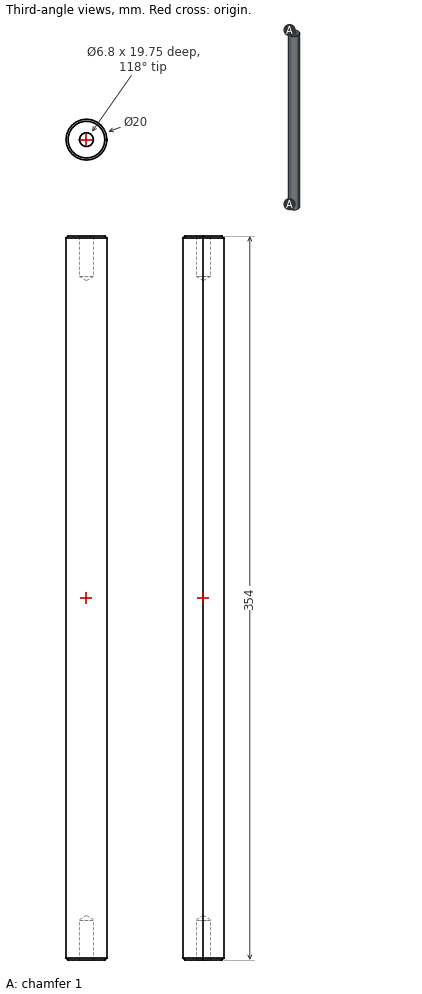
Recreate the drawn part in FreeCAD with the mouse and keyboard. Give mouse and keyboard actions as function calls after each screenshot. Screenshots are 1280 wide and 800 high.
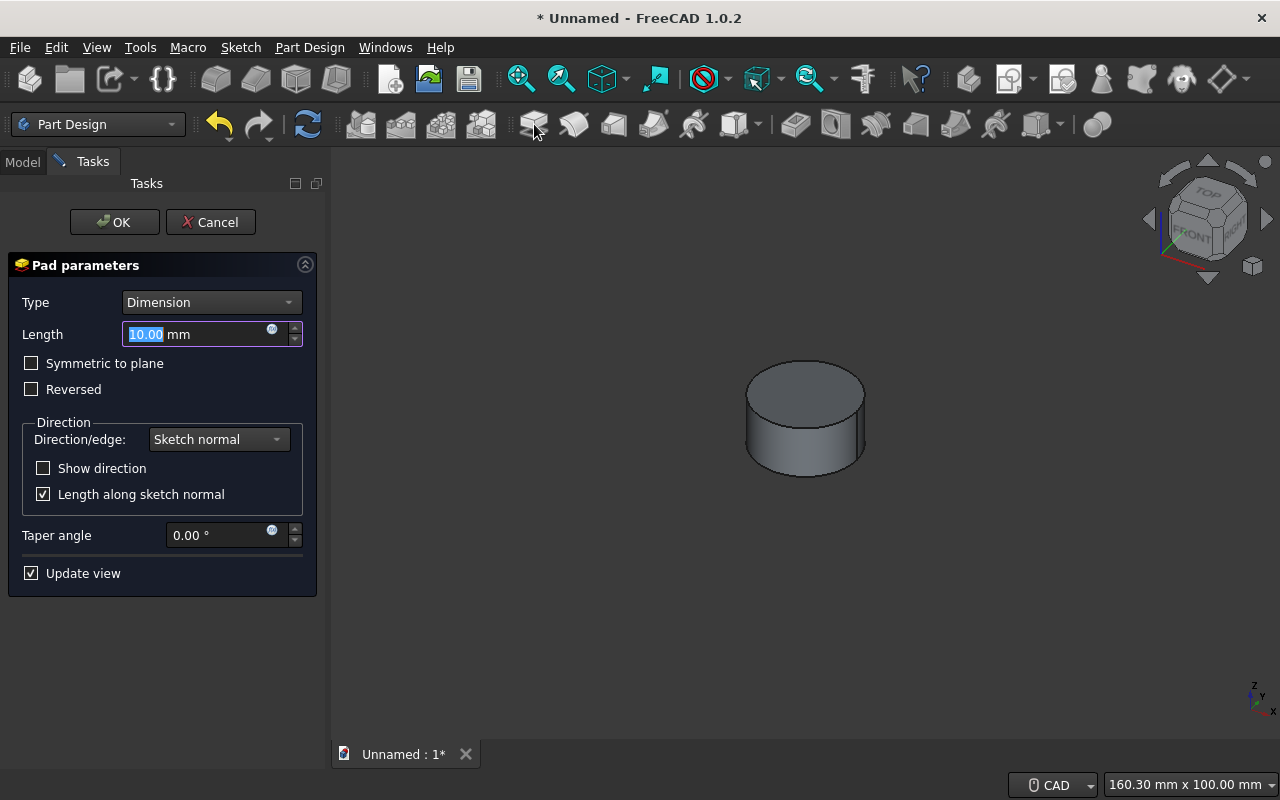
text(354)
key(Tab)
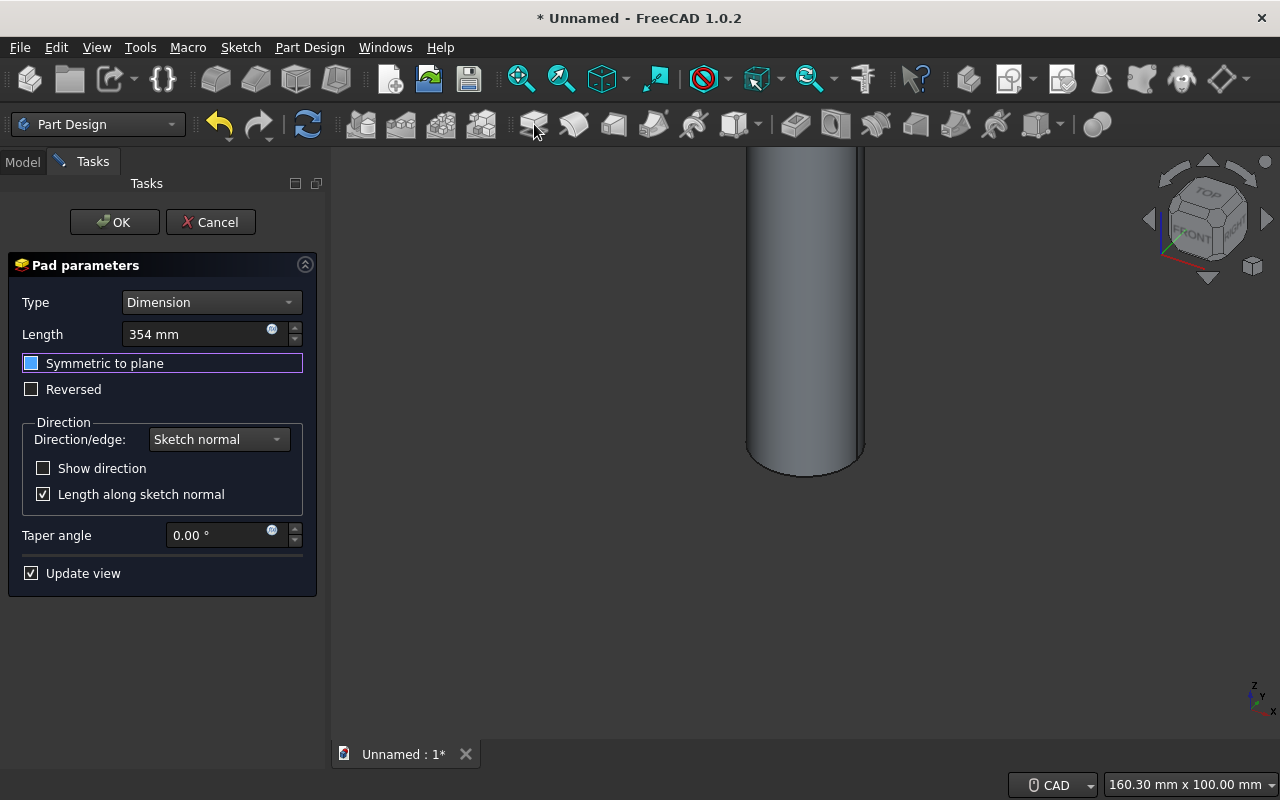
click(30, 363)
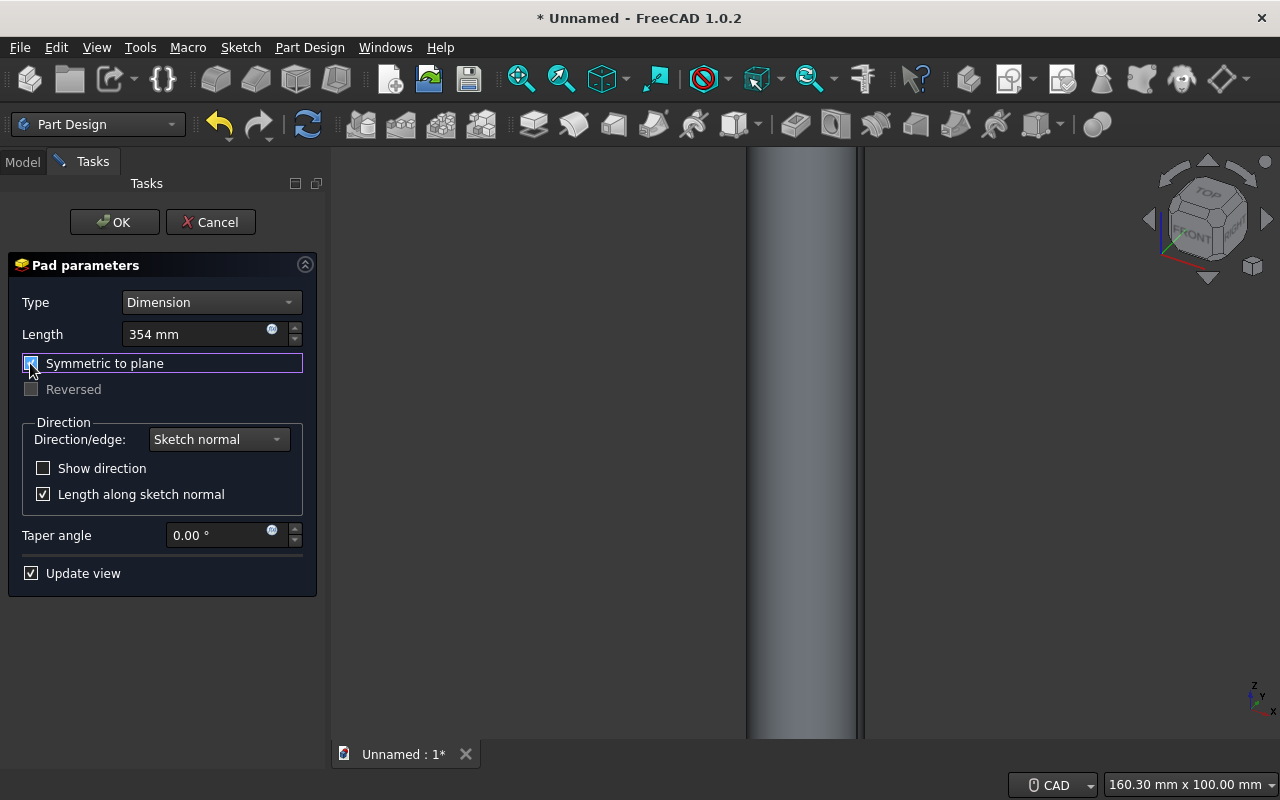
click(115, 222)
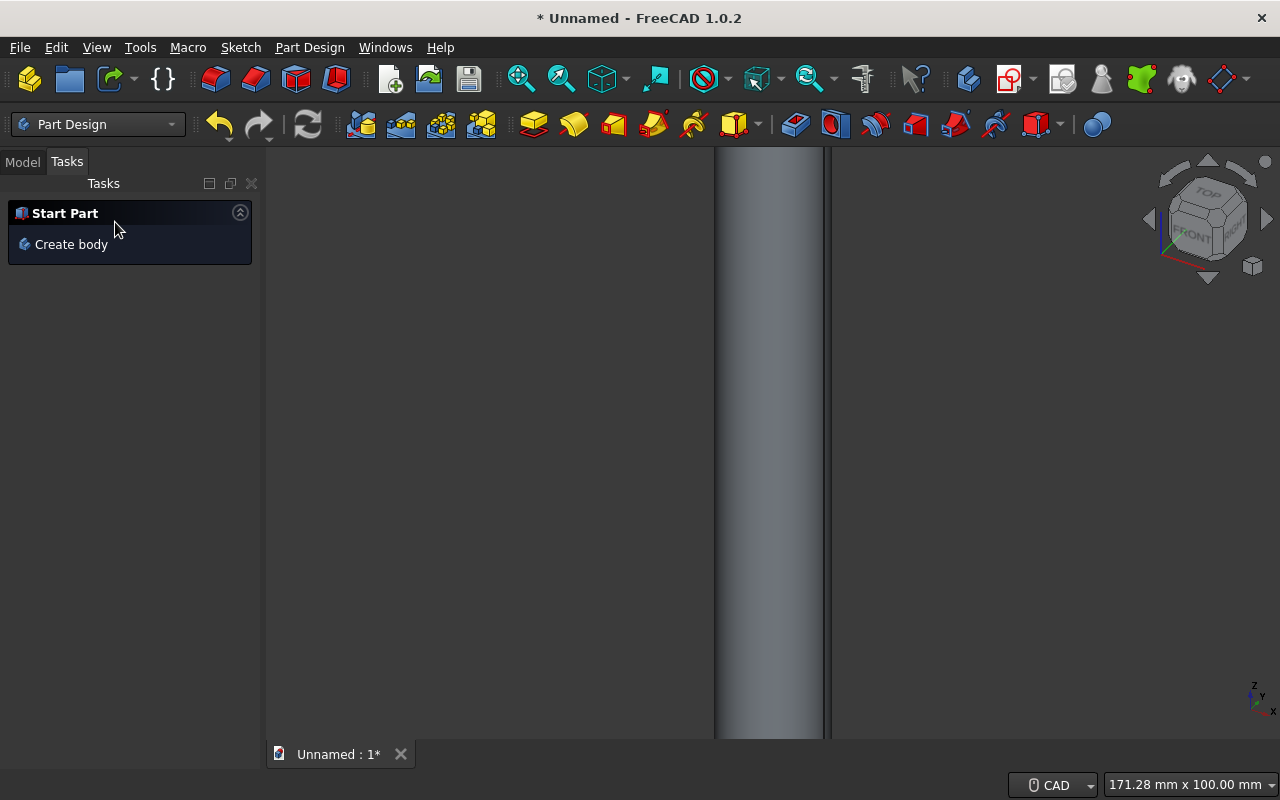
click(522, 80)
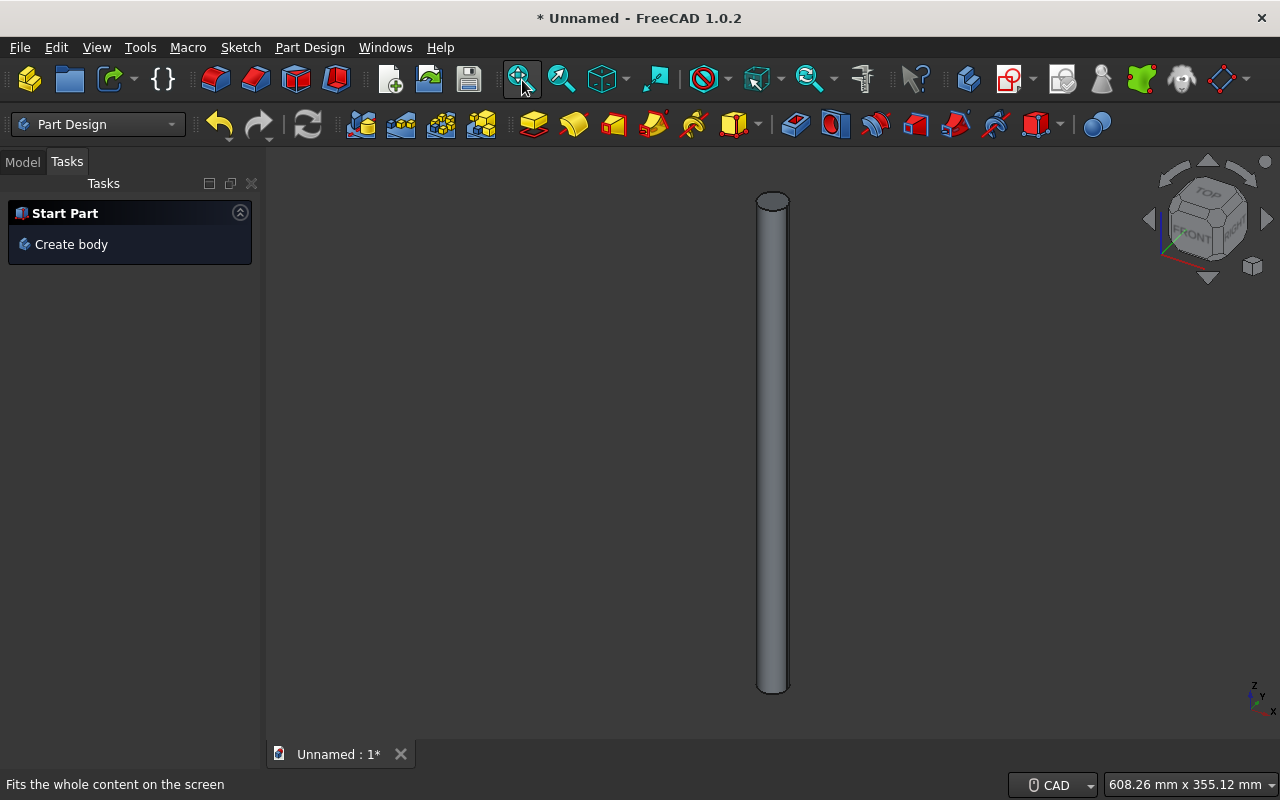
key(5)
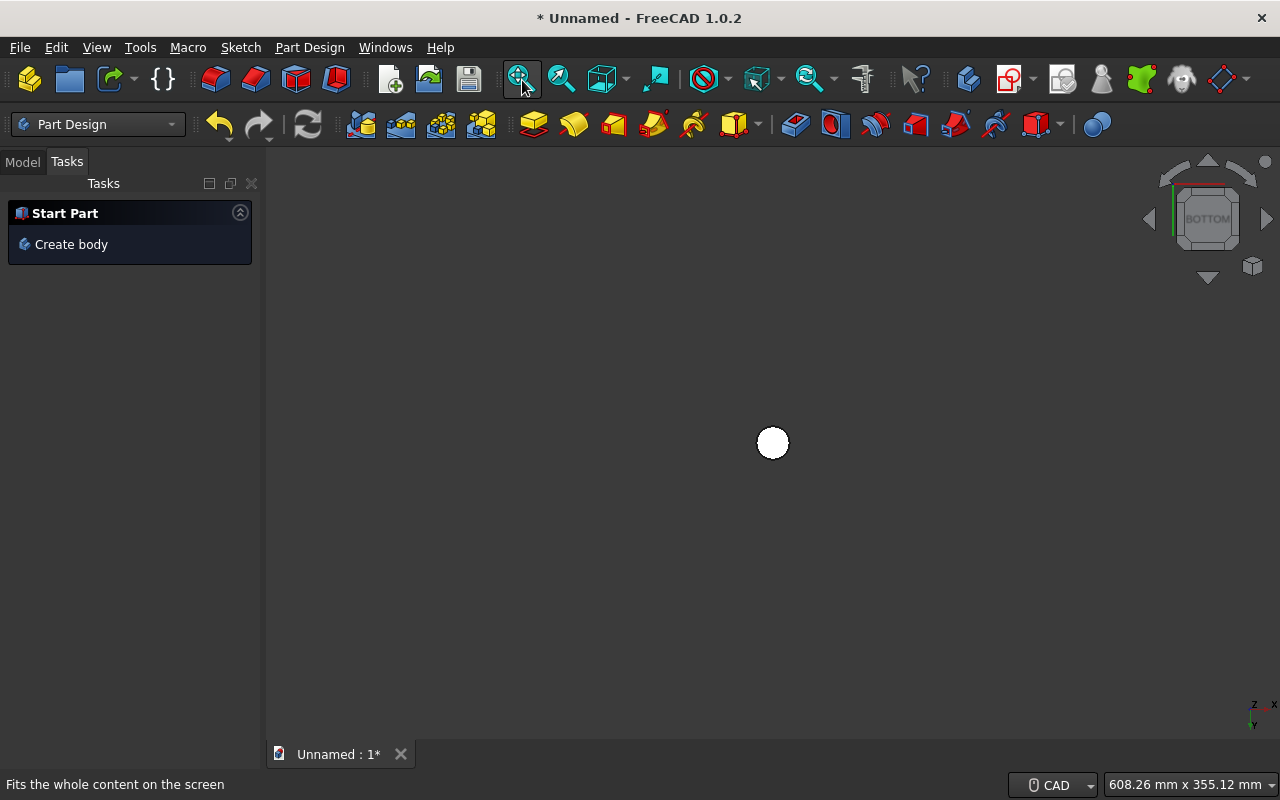
key(v)
key(f)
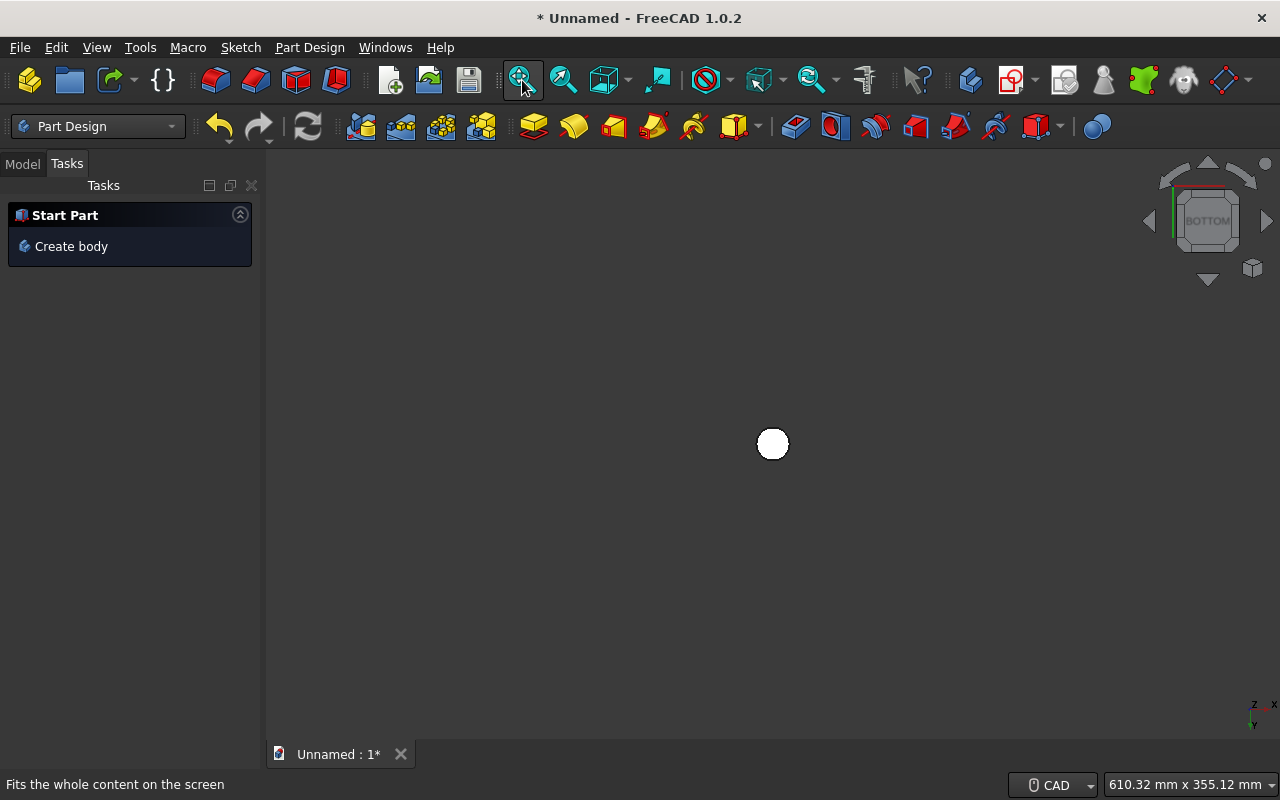
click(773, 443)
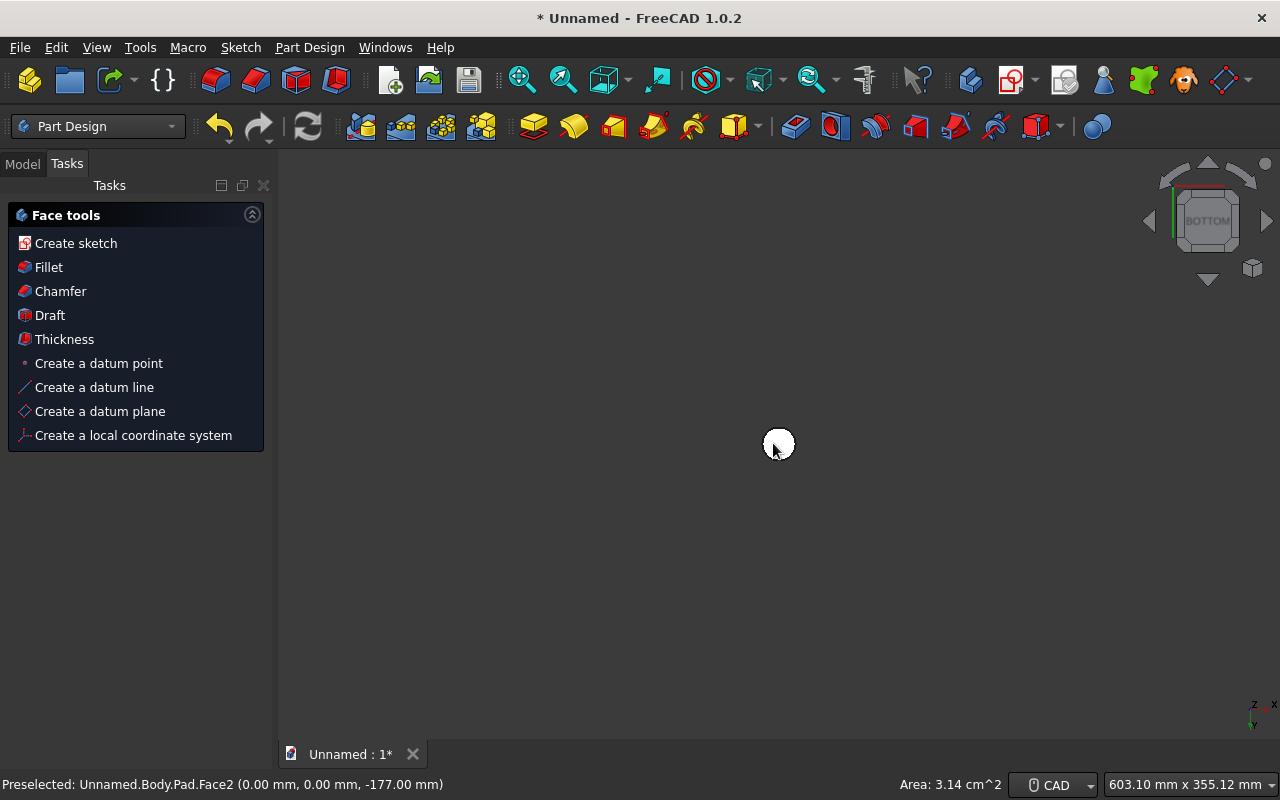
click(1012, 80)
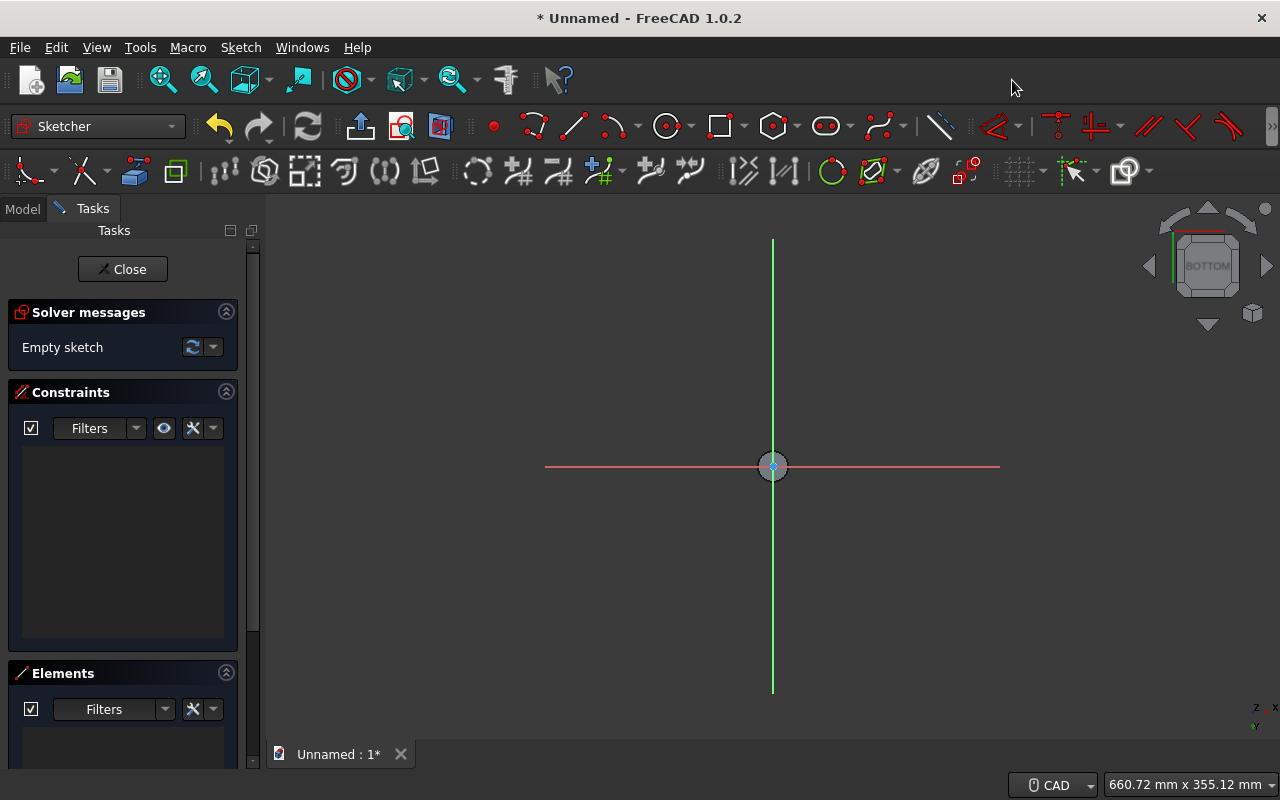
scroll(777, 466, up, 15)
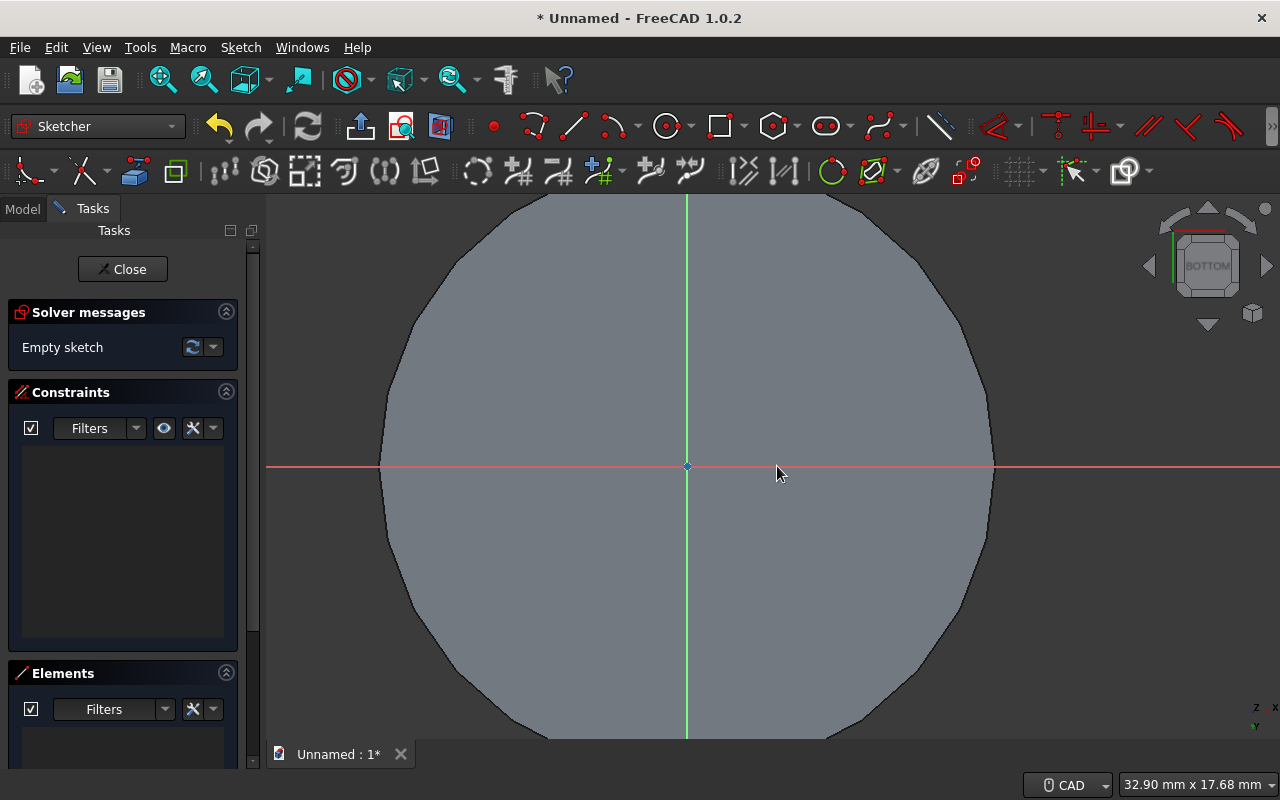
scroll(652, 467, up, 2)